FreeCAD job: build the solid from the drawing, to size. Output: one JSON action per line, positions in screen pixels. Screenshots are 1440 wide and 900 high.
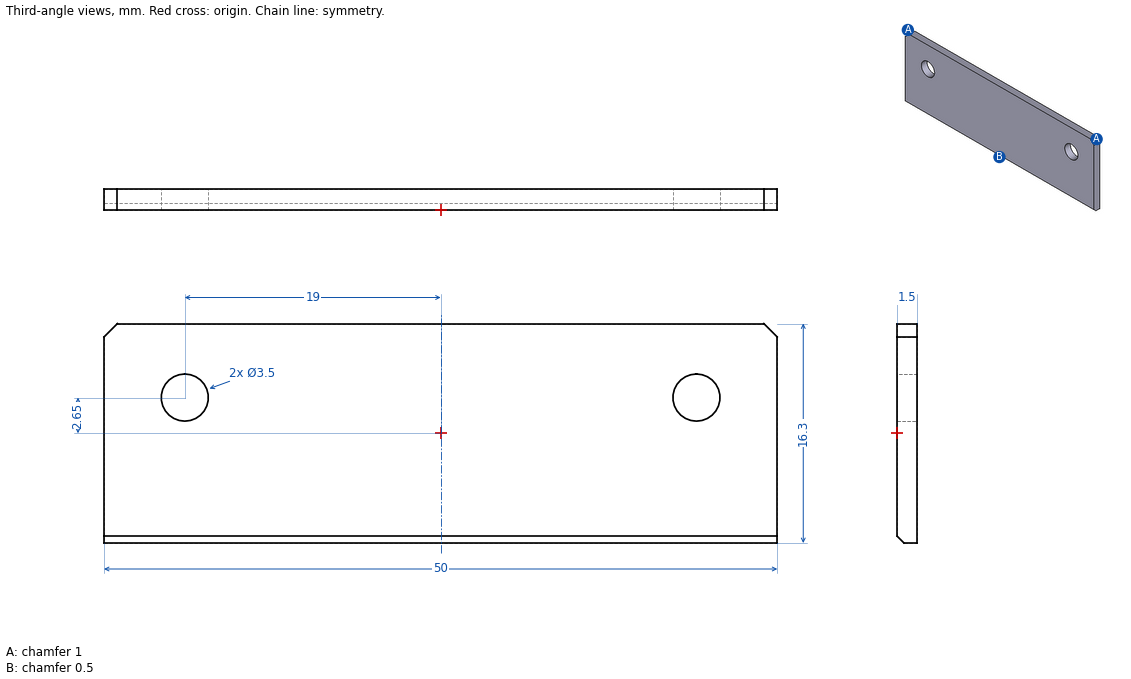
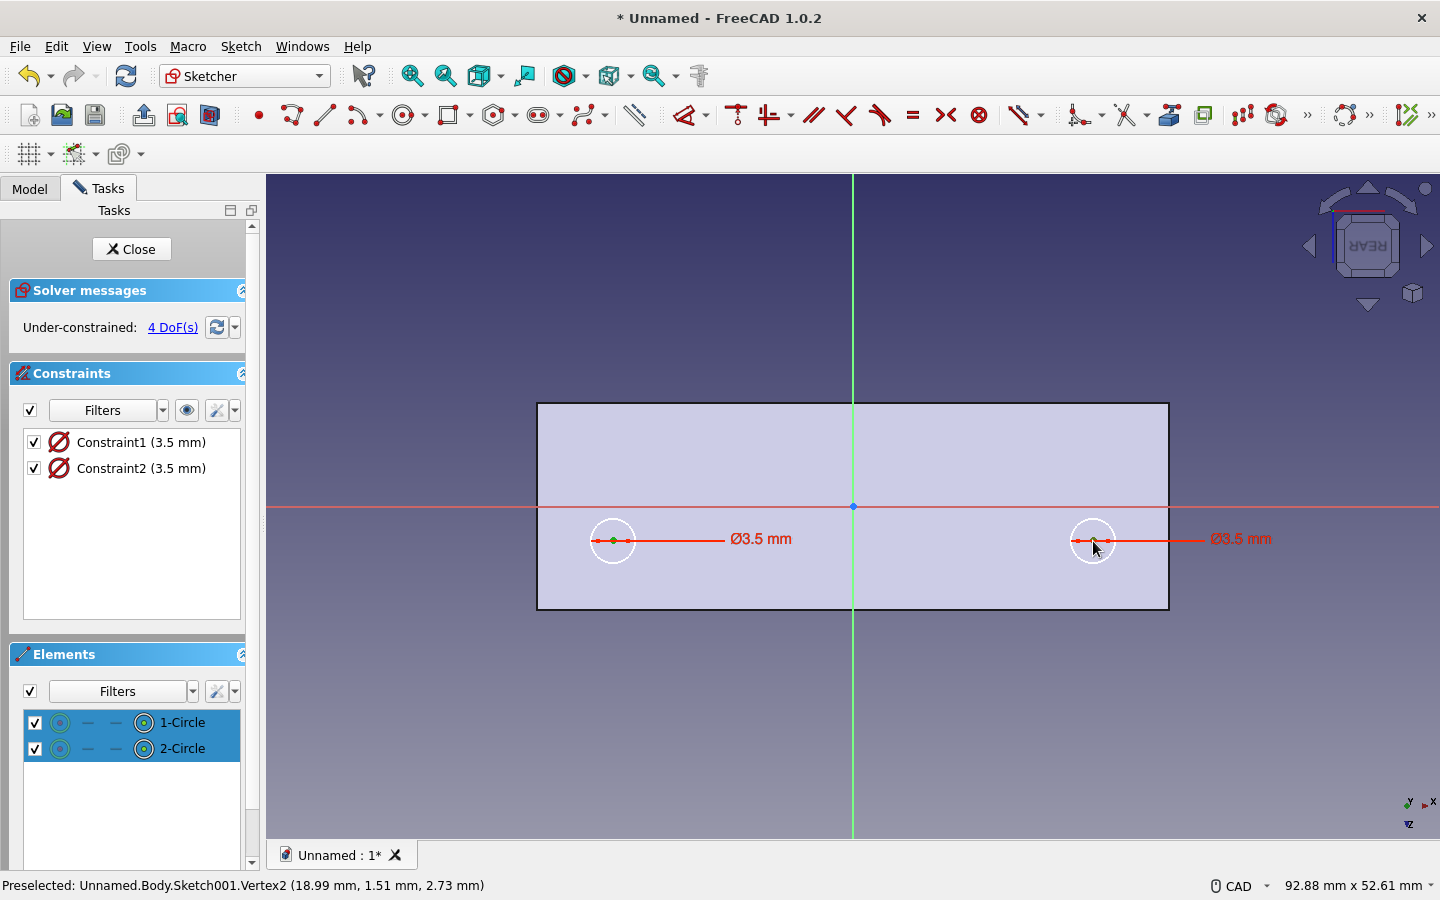
{"action": "left_click", "coordinate": [853, 768]}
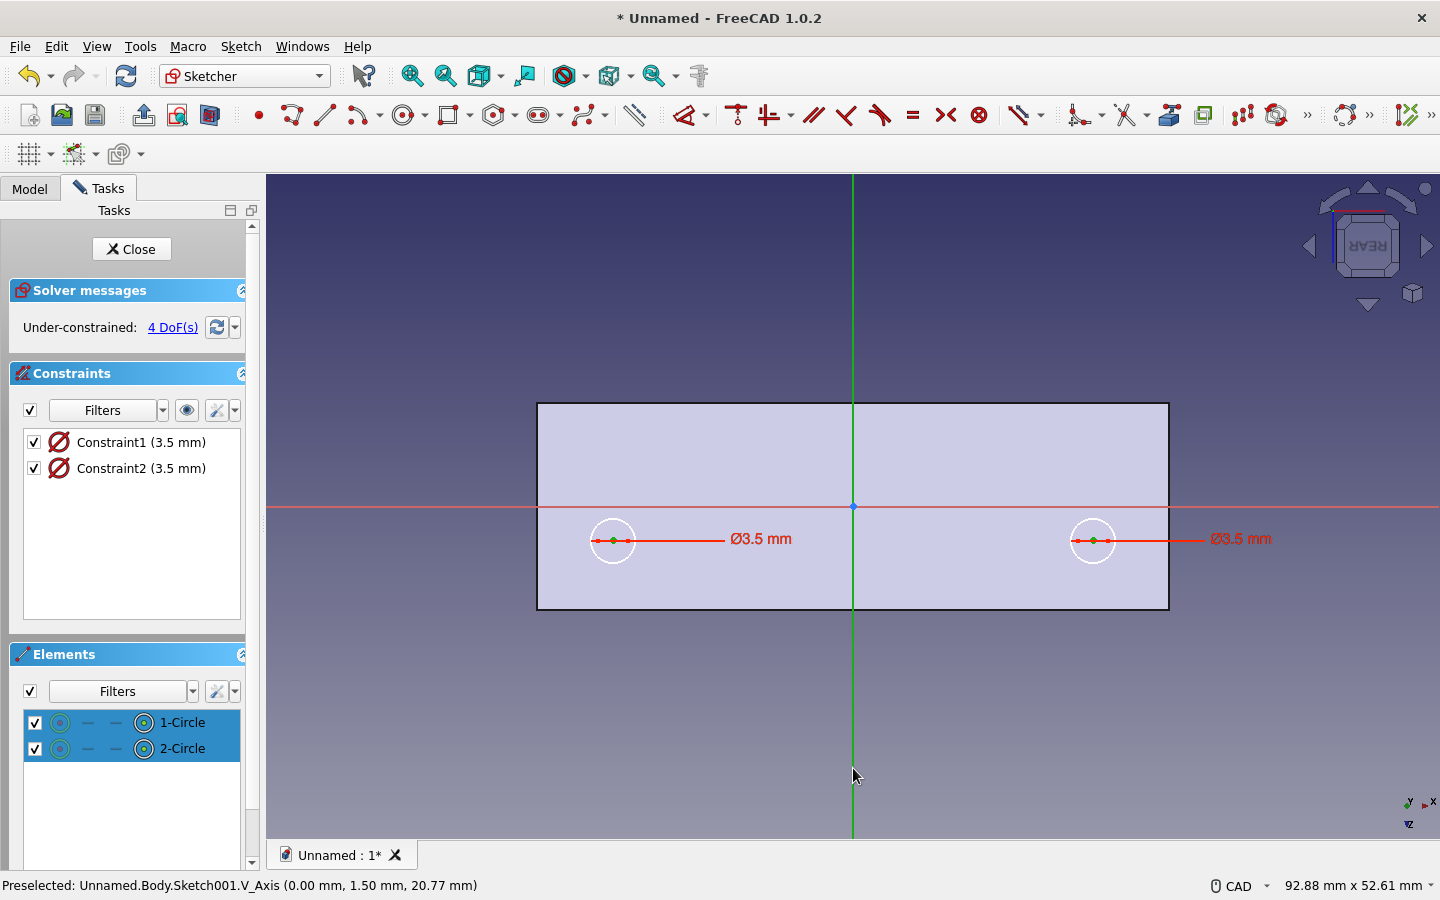
{"action": "key", "text": "s"}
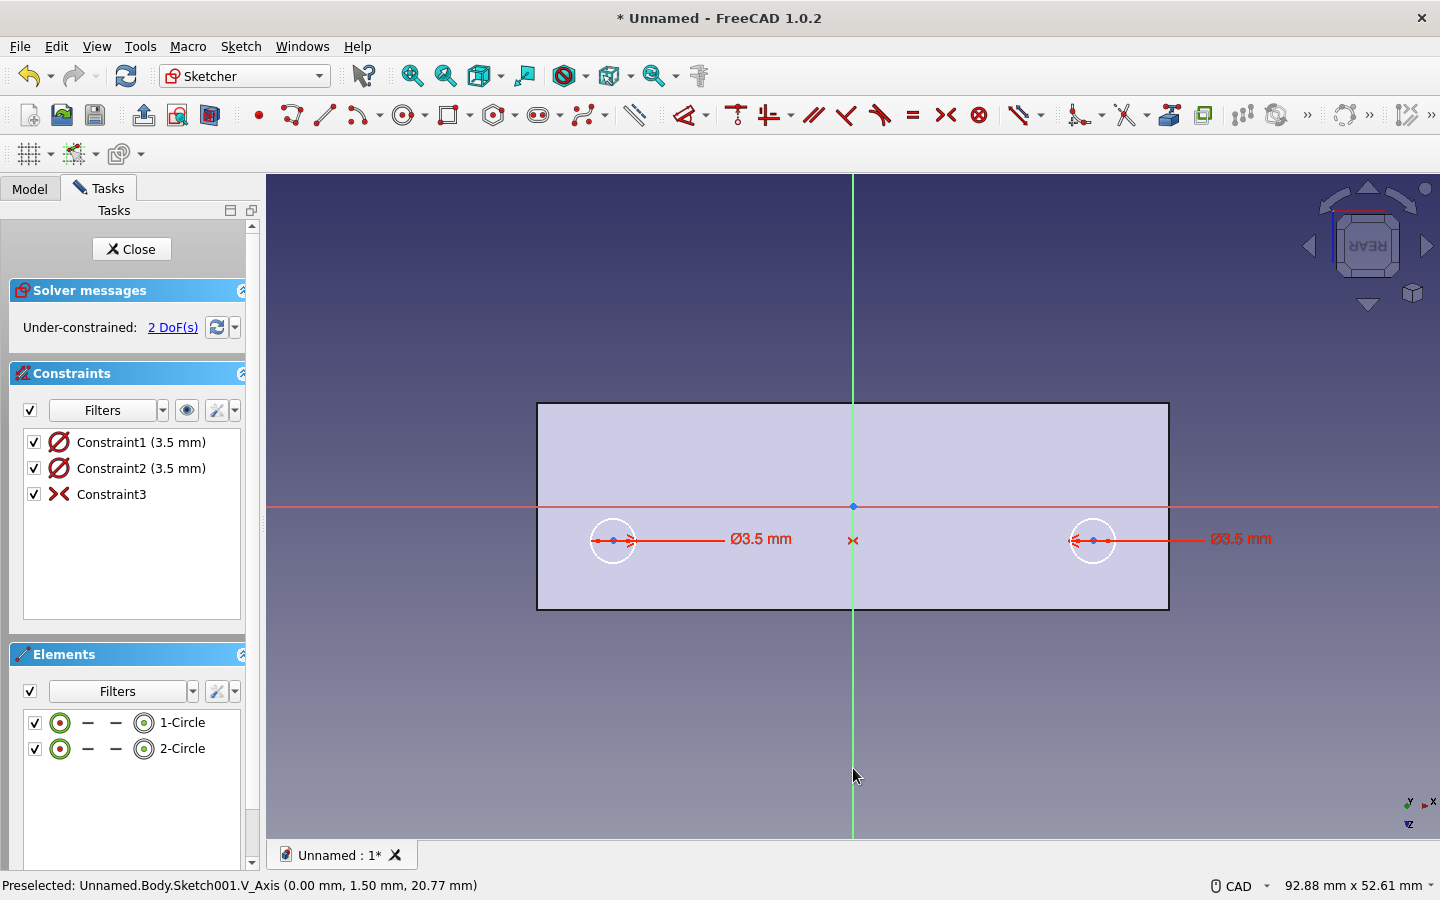
{"action": "key", "text": "d"}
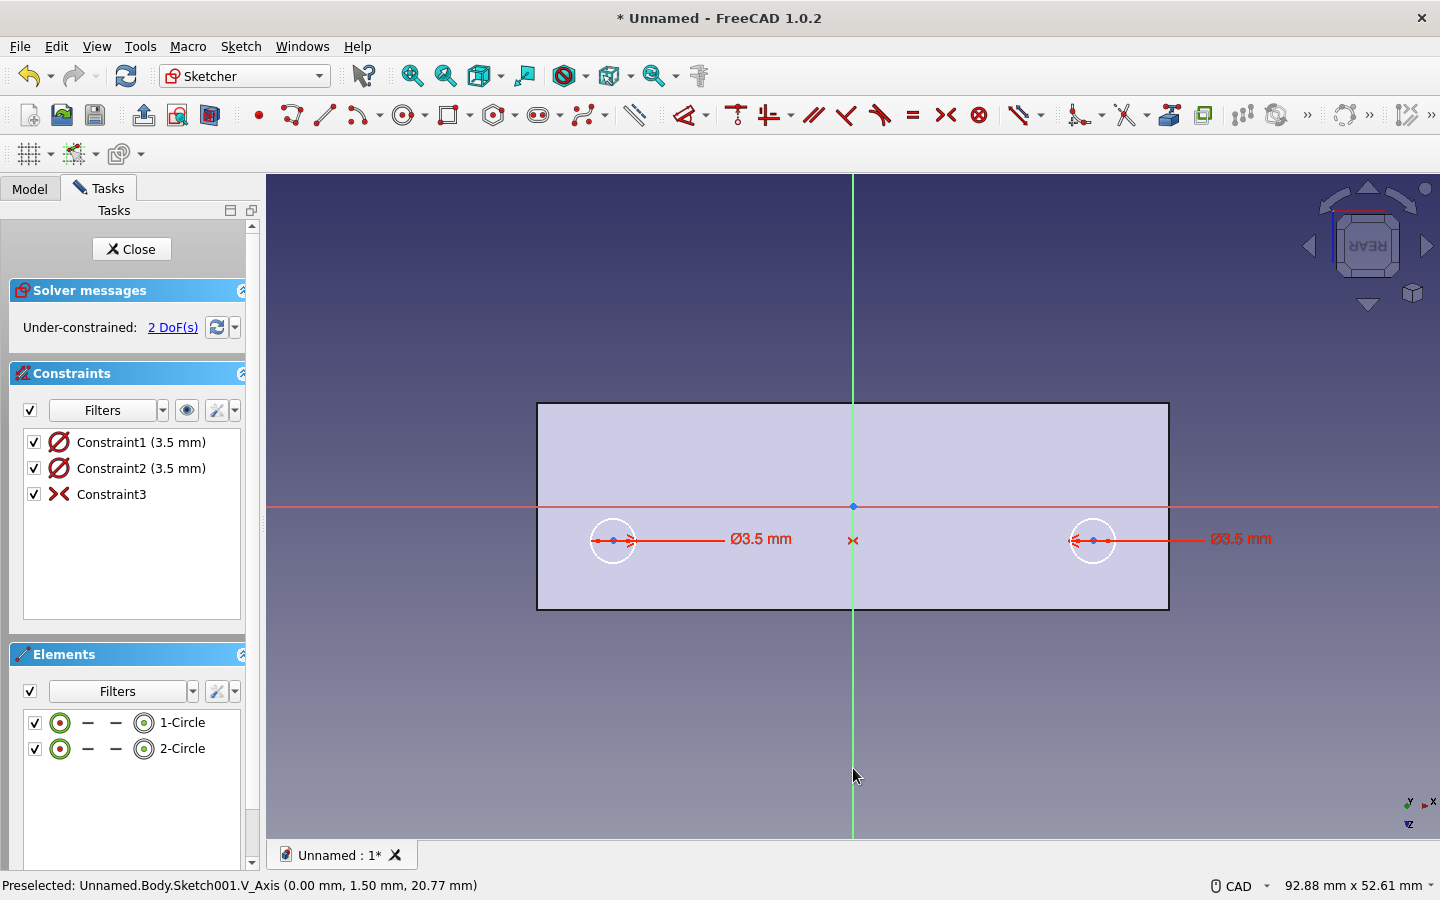
{"action": "left_click", "coordinate": [613, 541]}
{"action": "left_click", "coordinate": [733, 472]}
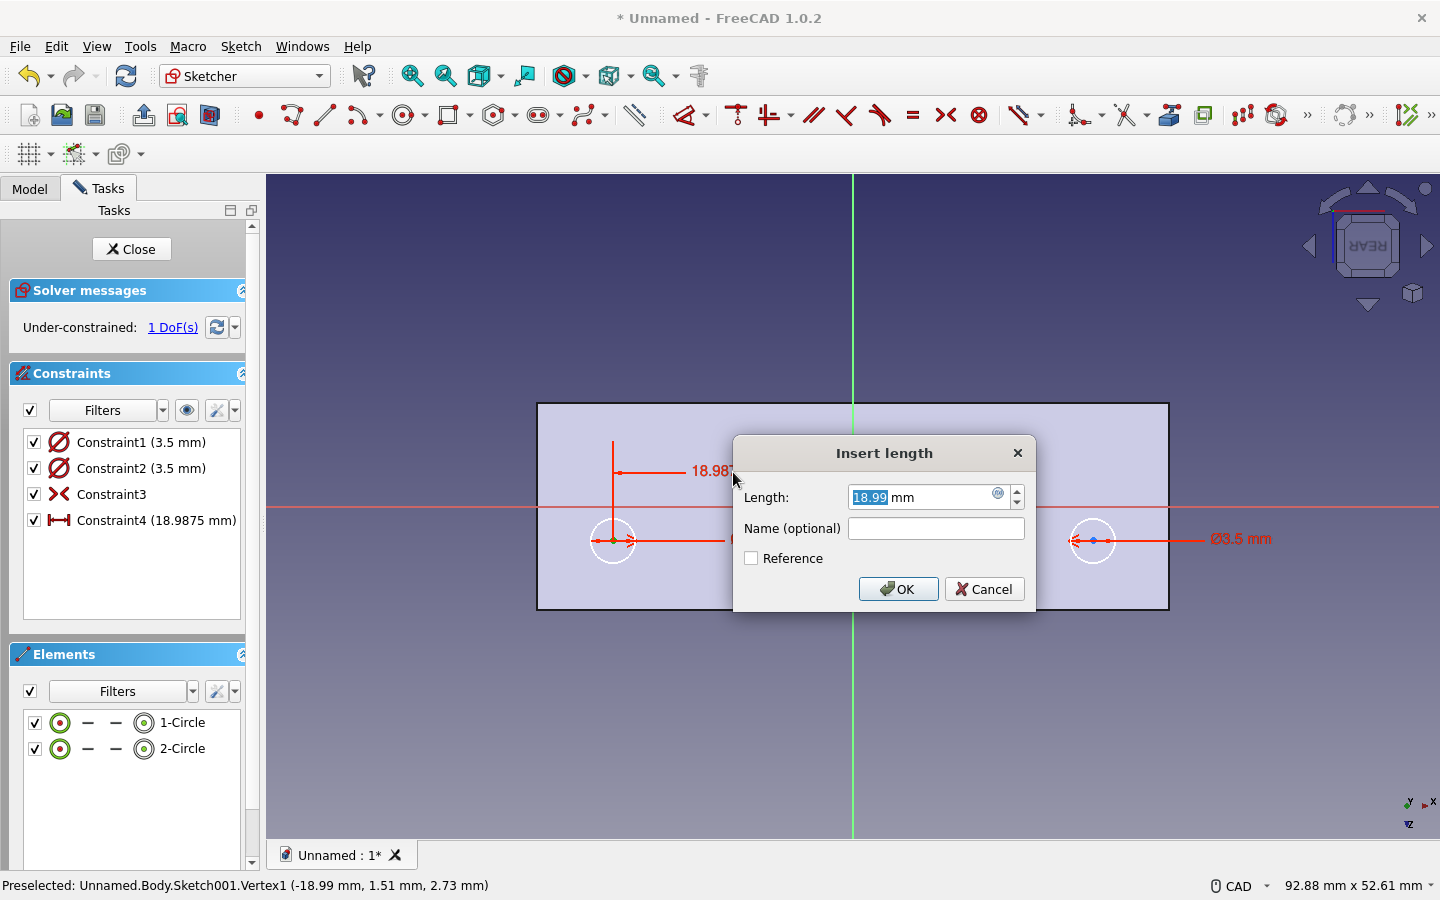
{"action": "type", "text": "19"}
{"action": "key", "text": "Return"}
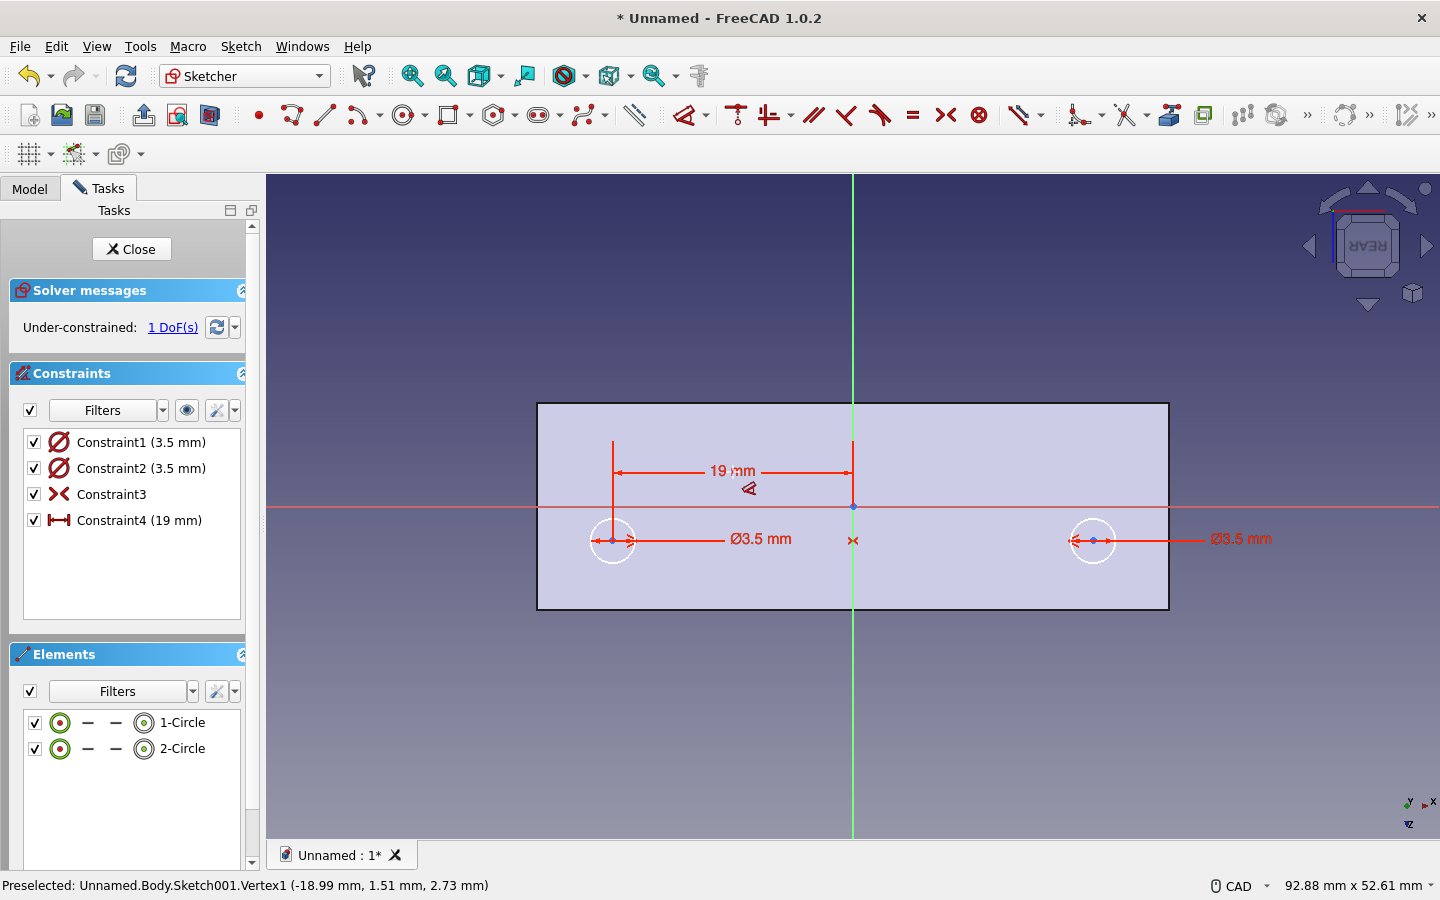
{"action": "left_click", "coordinate": [613, 541]}
{"action": "left_click", "coordinate": [579, 524]}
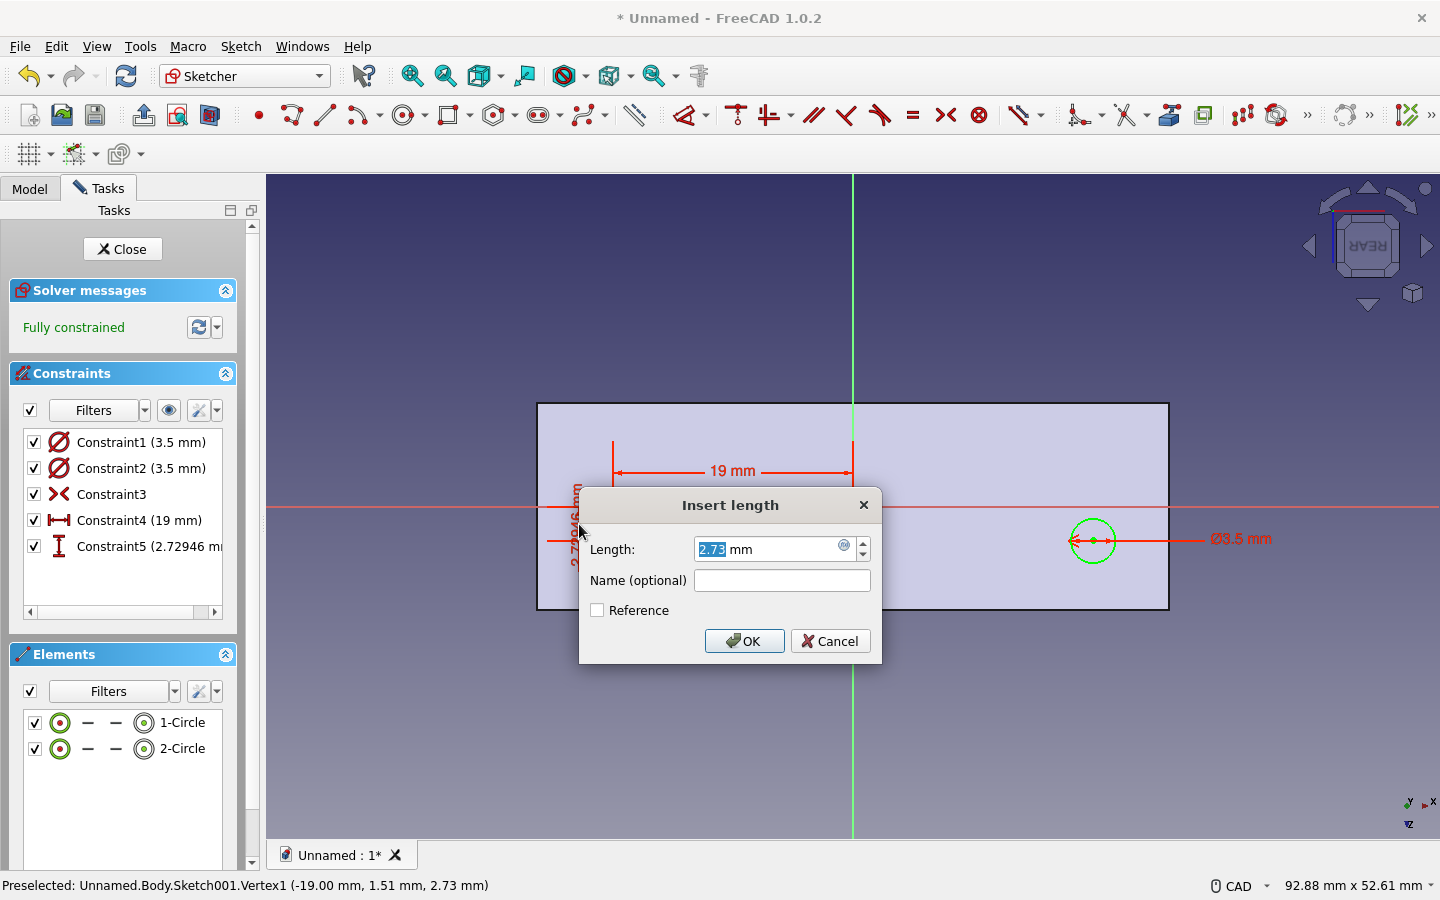
{"action": "type", "text": "2.65"}
{"action": "key", "text": "Return"}
{"action": "key", "text": "Escape"}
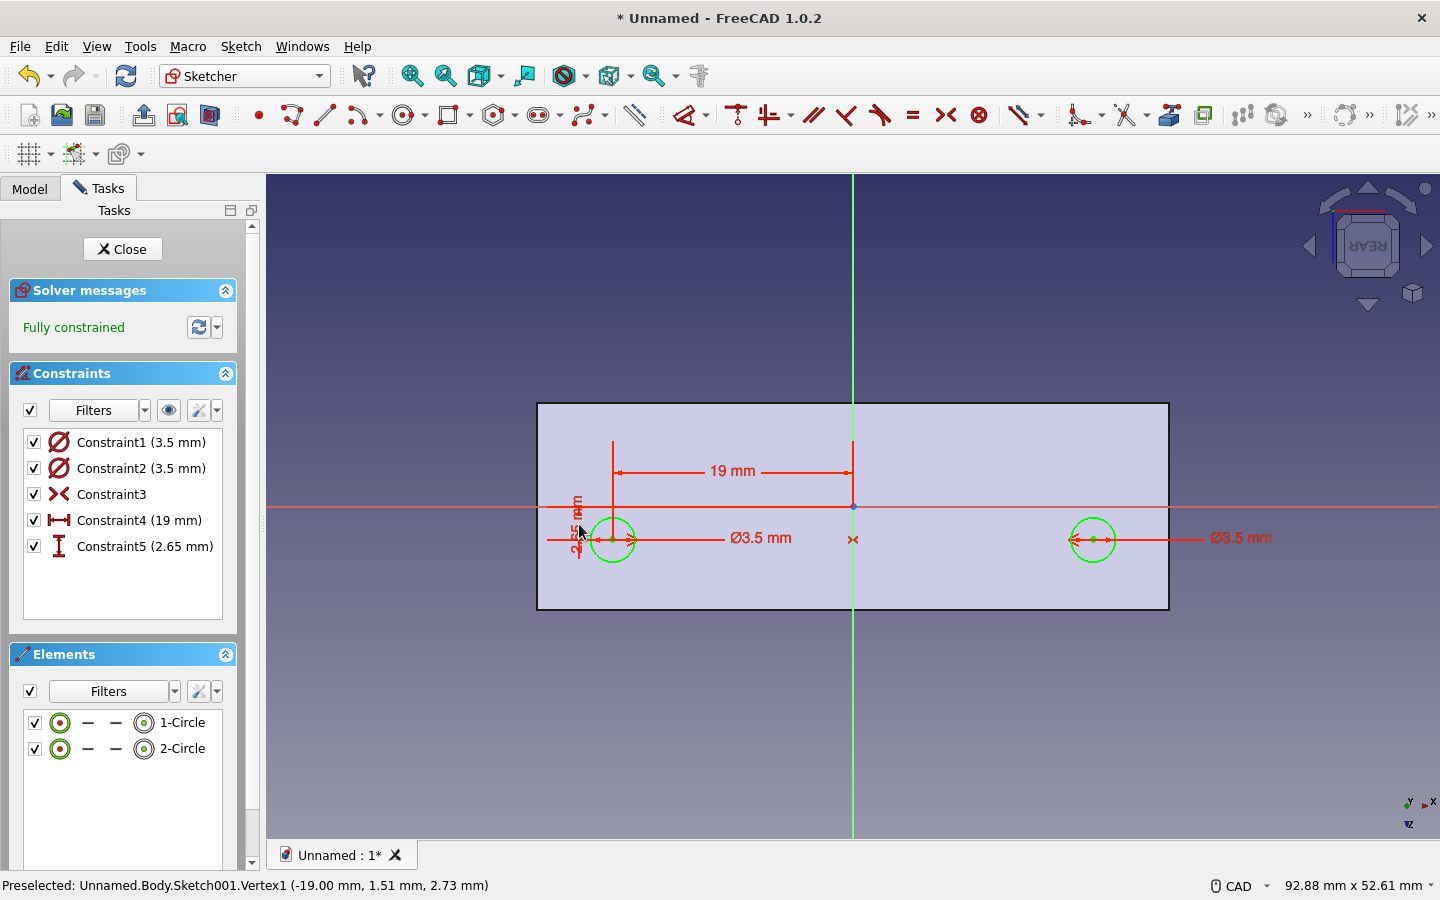
{"action": "left_click", "coordinate": [123, 249]}